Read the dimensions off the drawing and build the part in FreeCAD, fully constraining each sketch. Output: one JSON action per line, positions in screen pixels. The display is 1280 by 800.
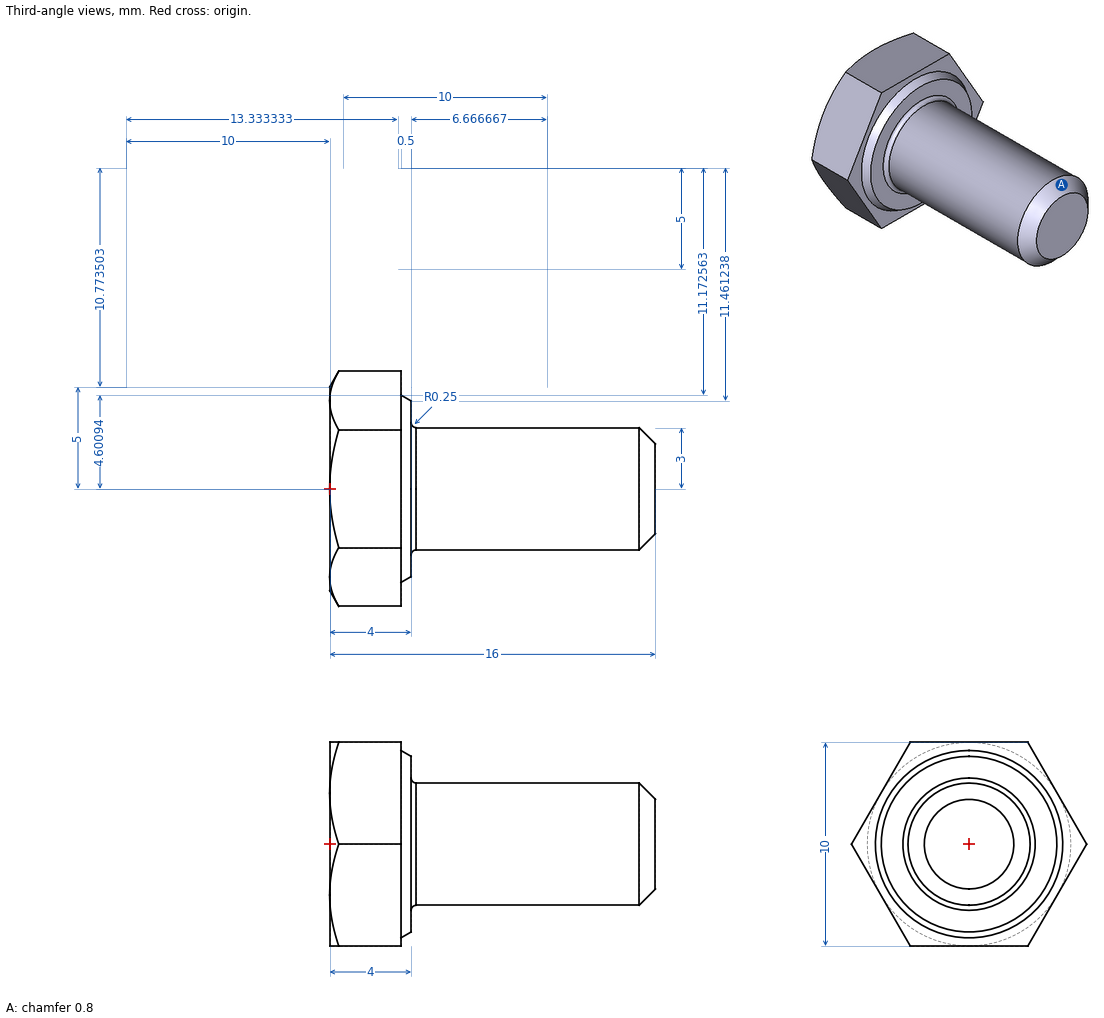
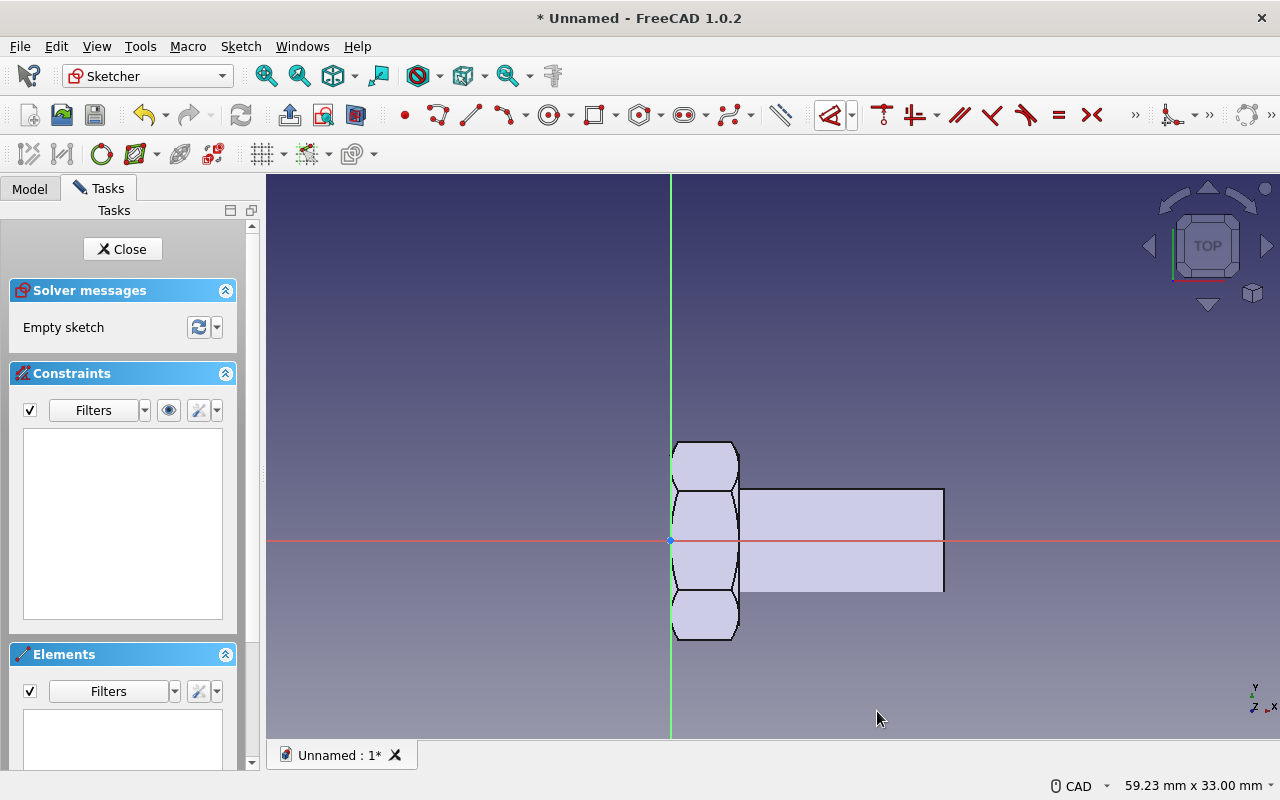
{"action": "left_click", "coordinate": [438, 116]}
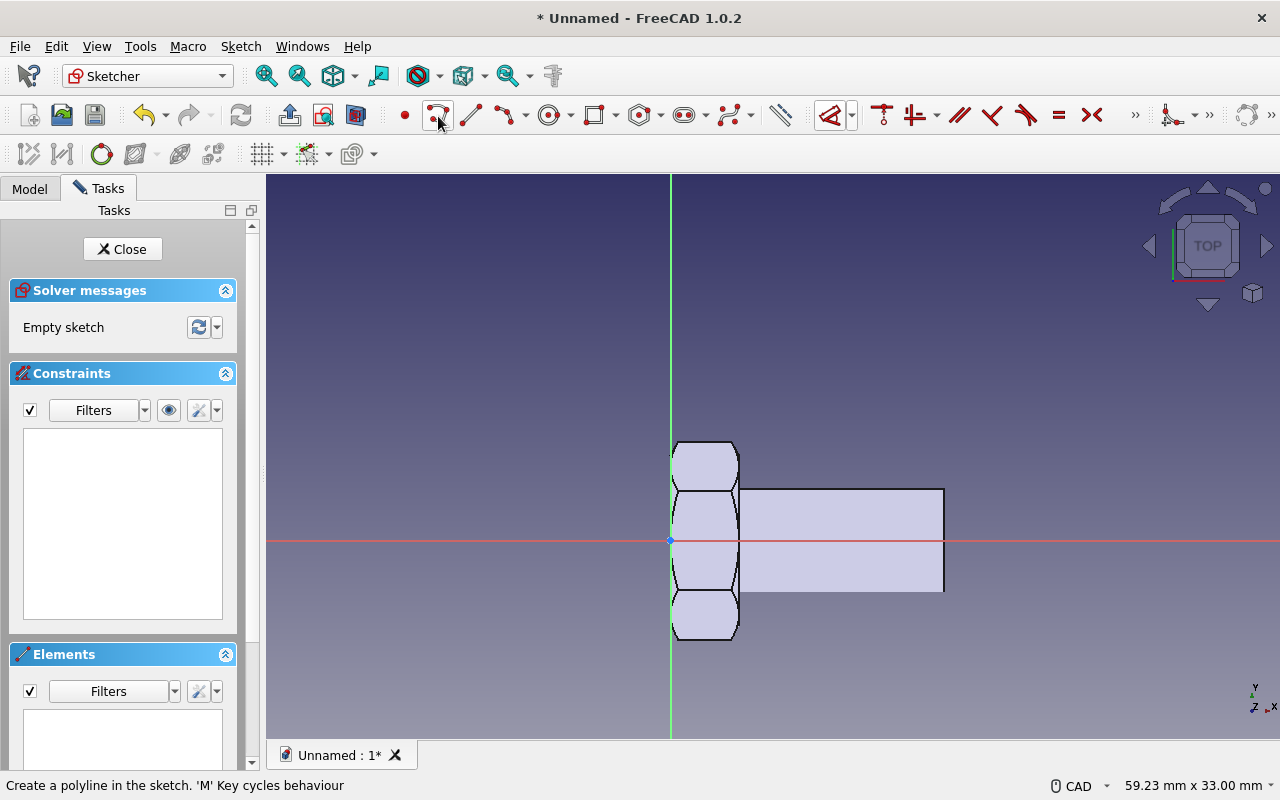
{"action": "left_click", "coordinate": [730, 462]}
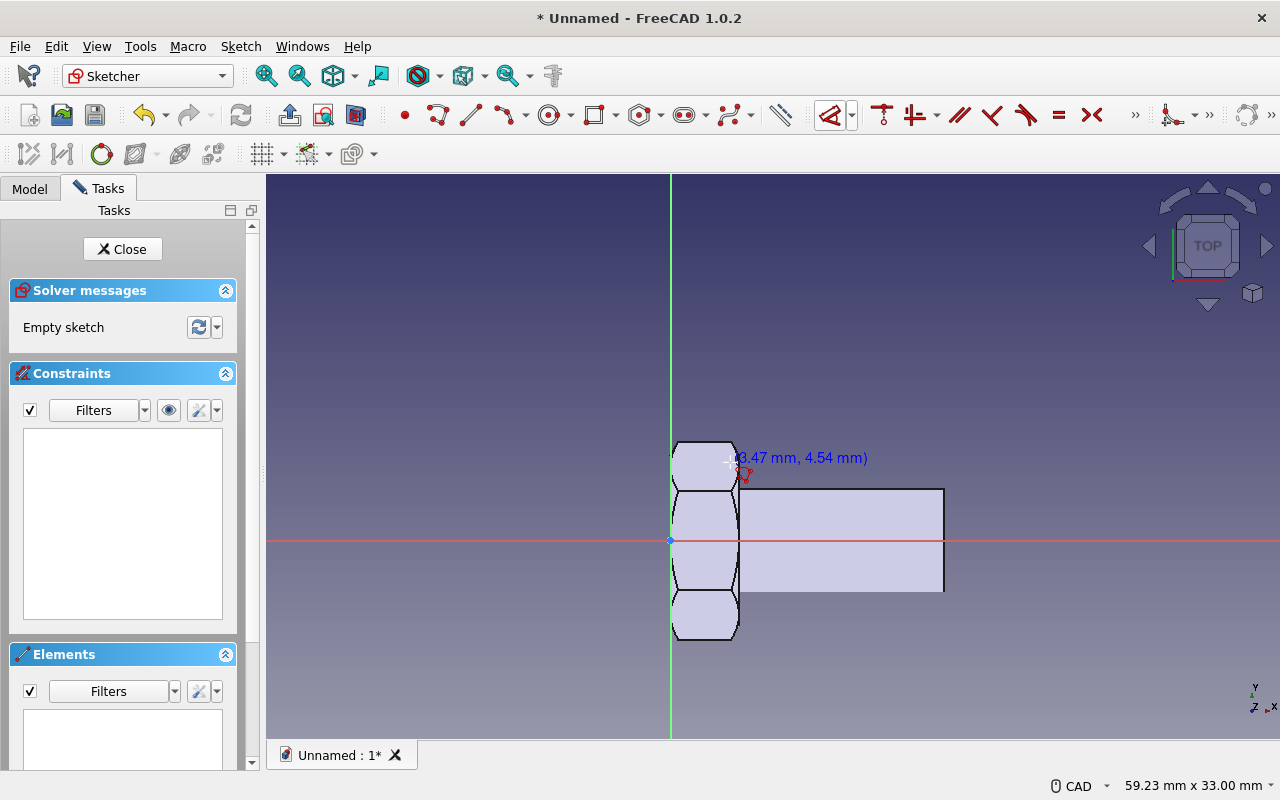
{"action": "scroll", "coordinate": [739, 467], "scroll_direction": "up", "scroll_amount": 3}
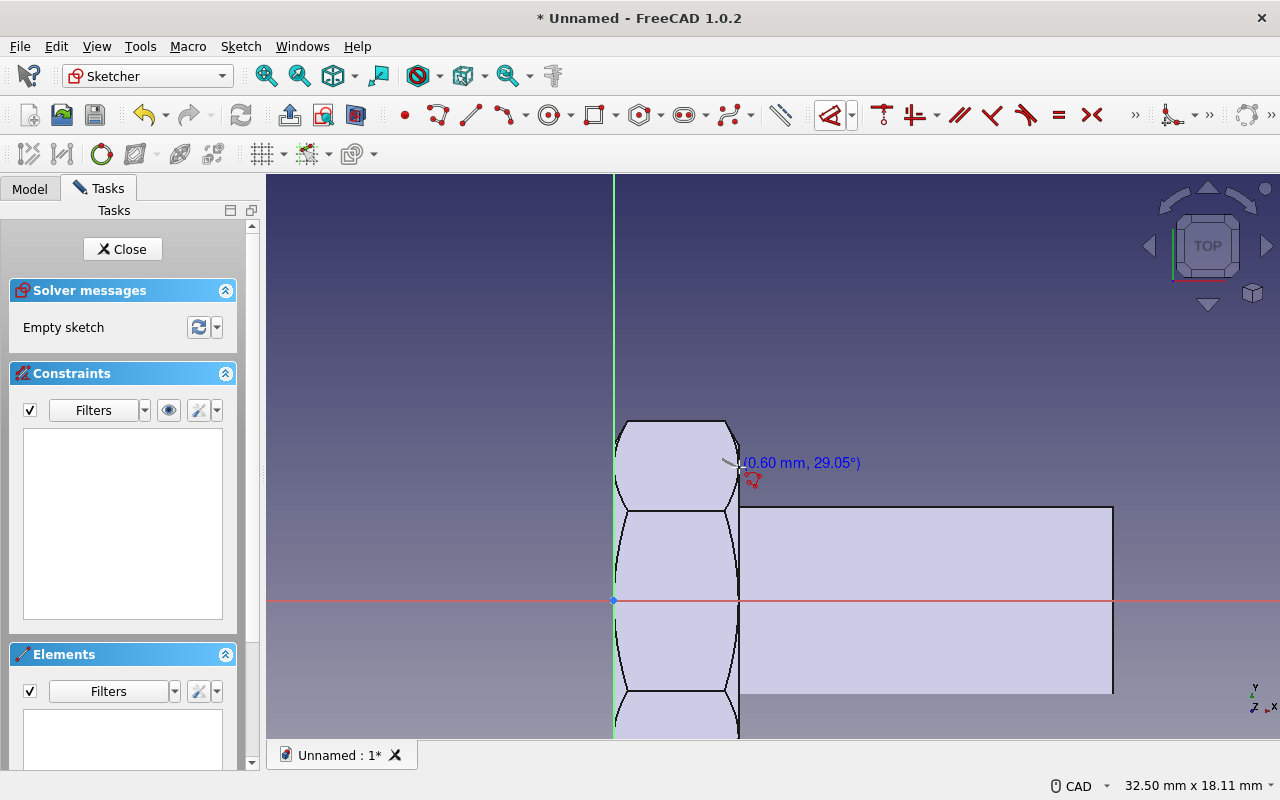
{"action": "left_click", "coordinate": [739, 466]}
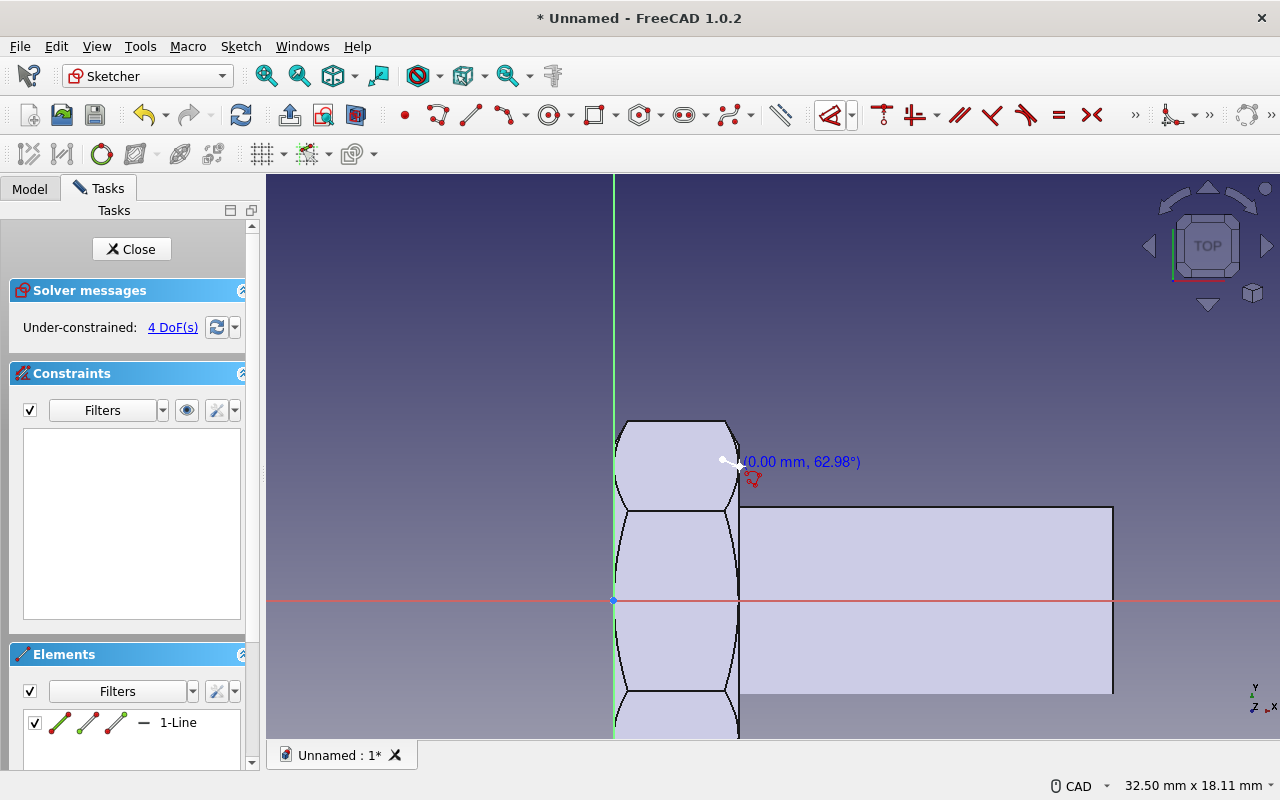
{"action": "scroll", "coordinate": [762, 663], "scroll_direction": "down", "scroll_amount": 2}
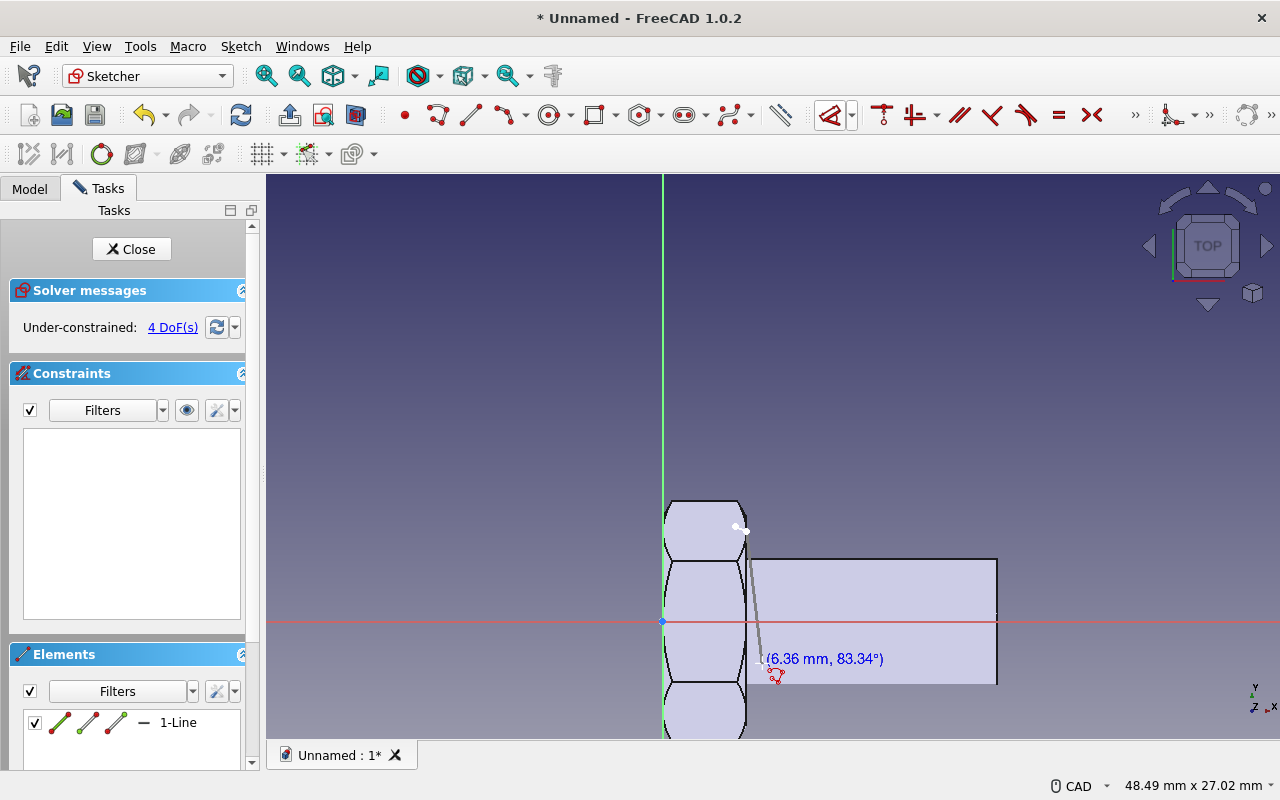
{"action": "left_click", "coordinate": [747, 292]}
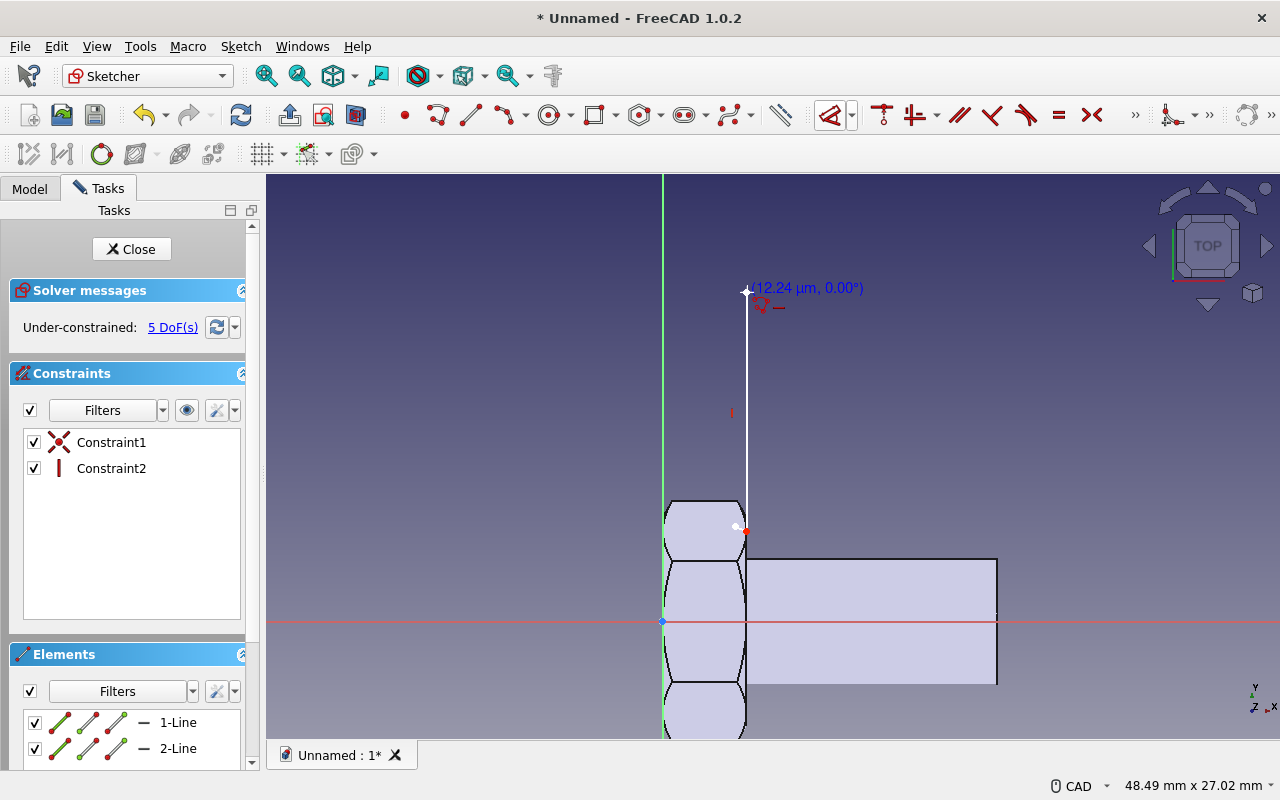
{"action": "scroll", "coordinate": [736, 292], "scroll_direction": "up", "scroll_amount": 3}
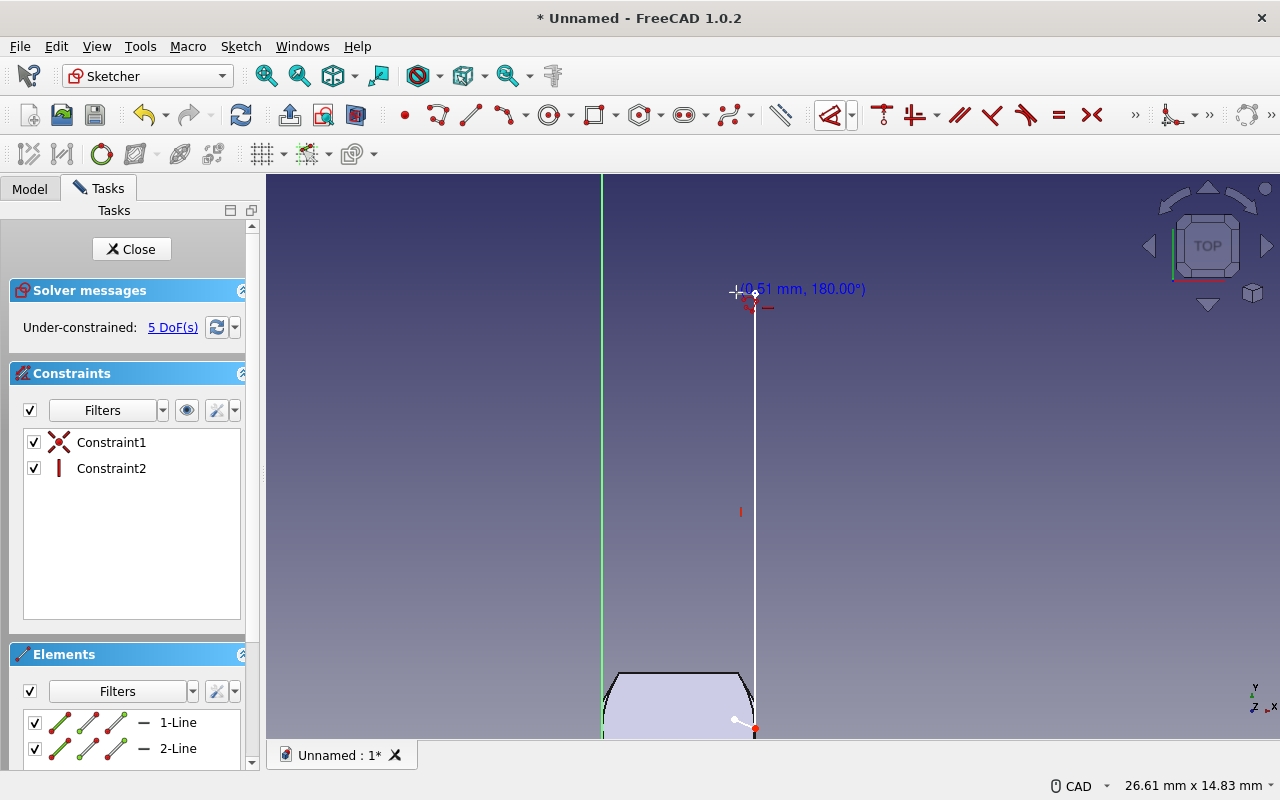
{"action": "left_click", "coordinate": [736, 292]}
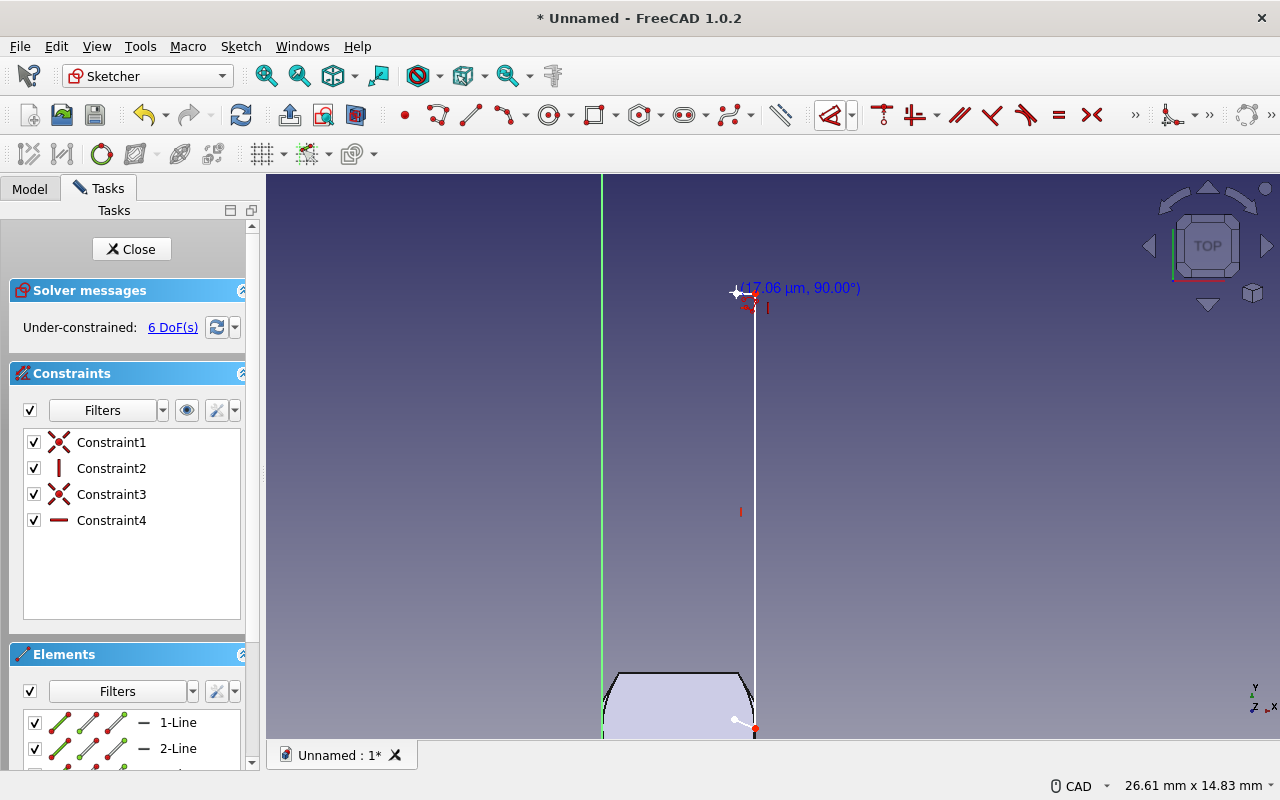
{"action": "scroll", "coordinate": [736, 292], "scroll_direction": "down", "scroll_amount": 3}